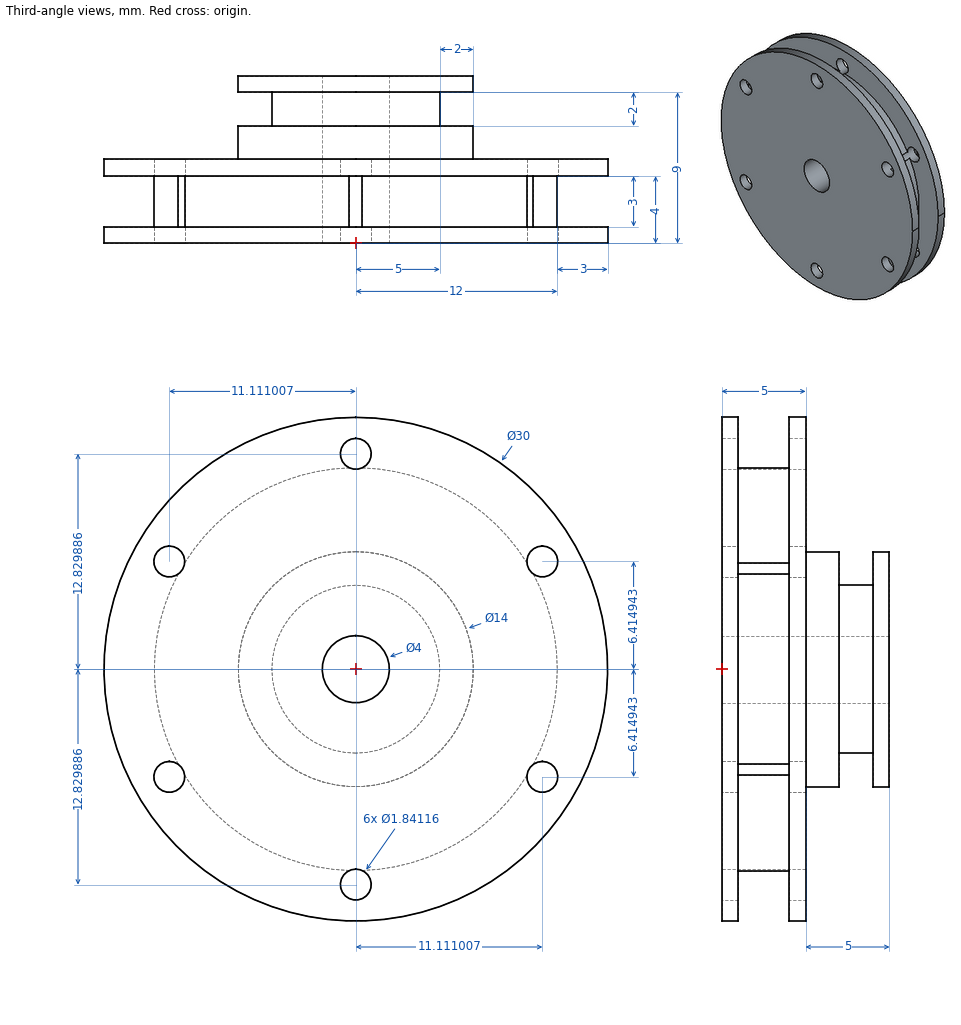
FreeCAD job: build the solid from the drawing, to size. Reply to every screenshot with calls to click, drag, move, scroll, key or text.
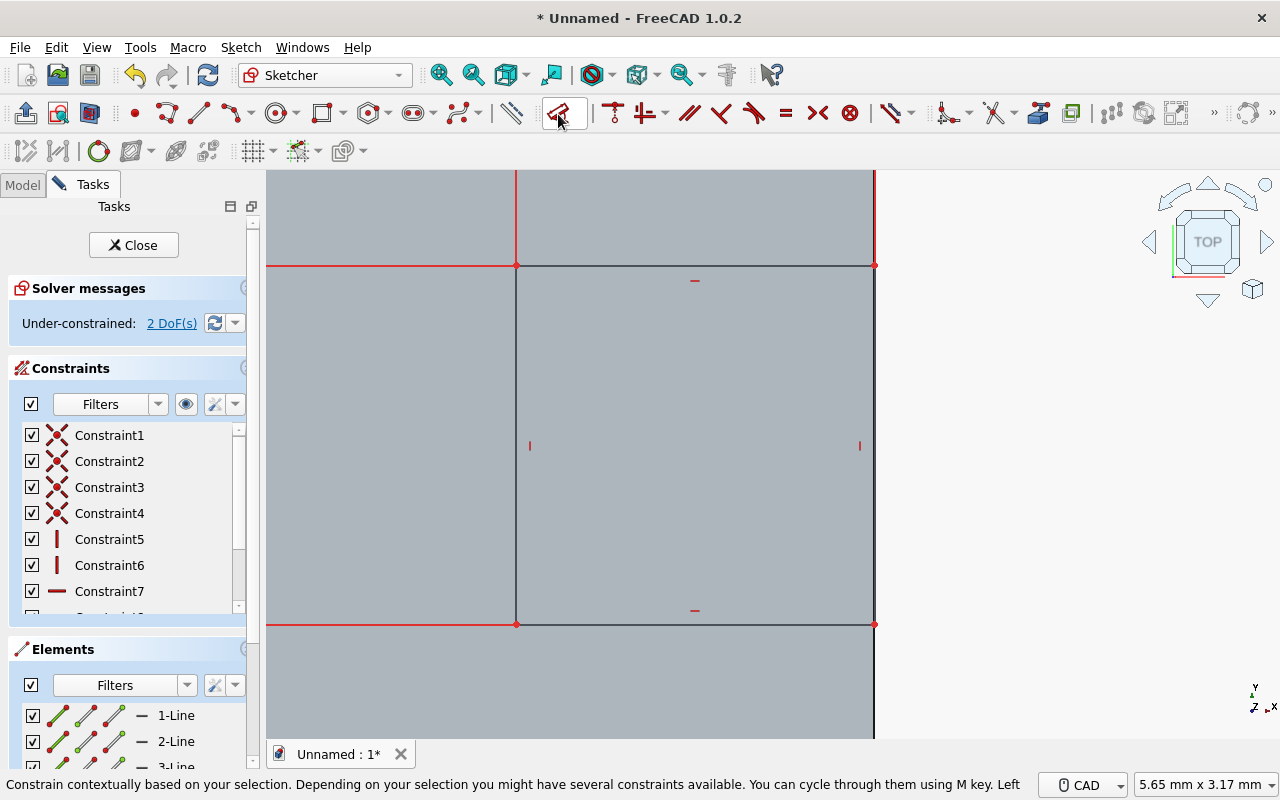
click(516, 266)
click(405, 232)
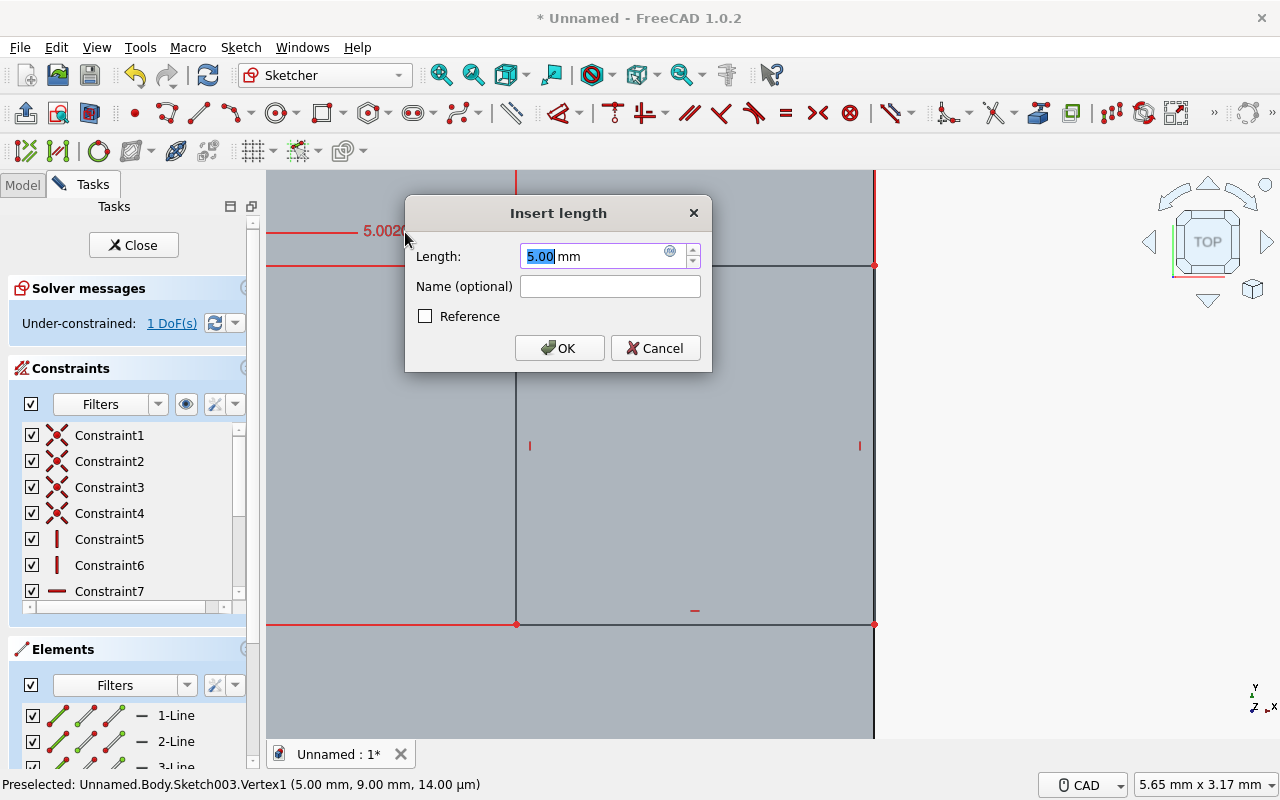
text(5)
key(Return)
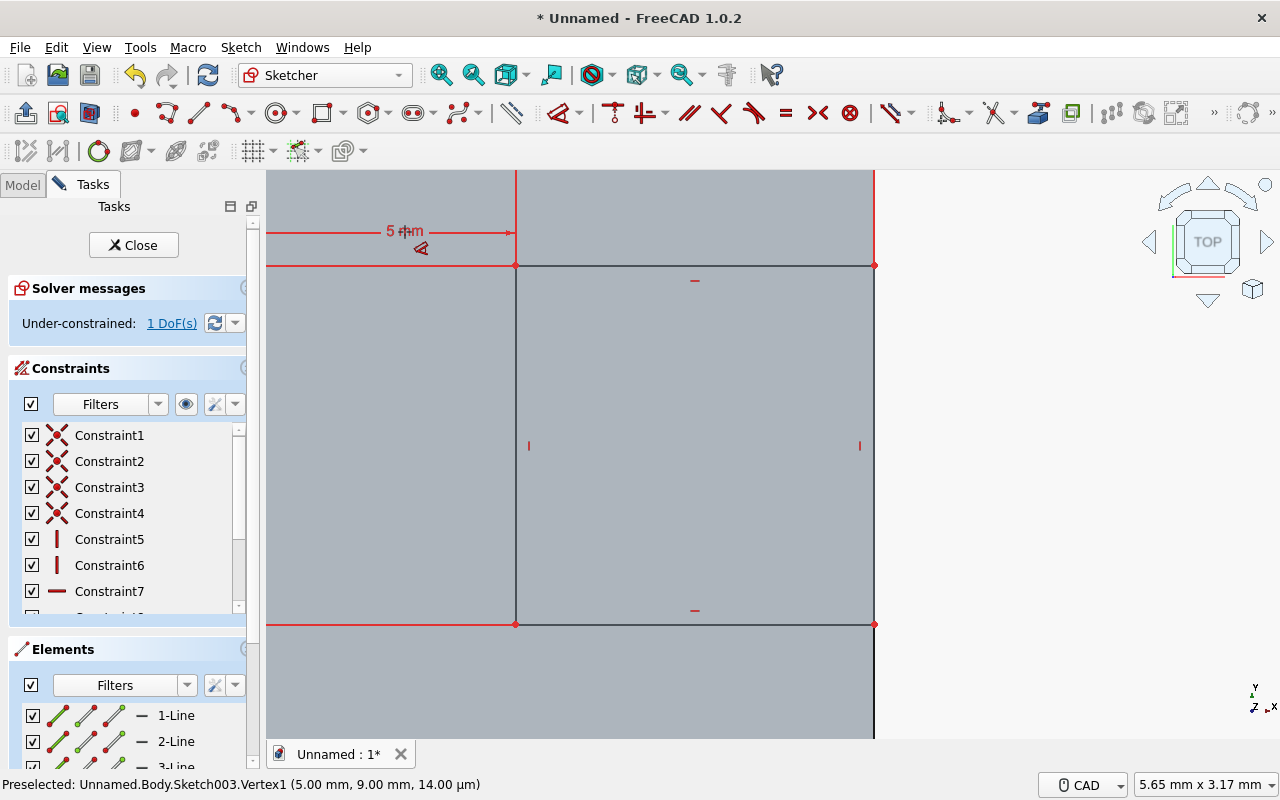
click(516, 266)
click(550, 489)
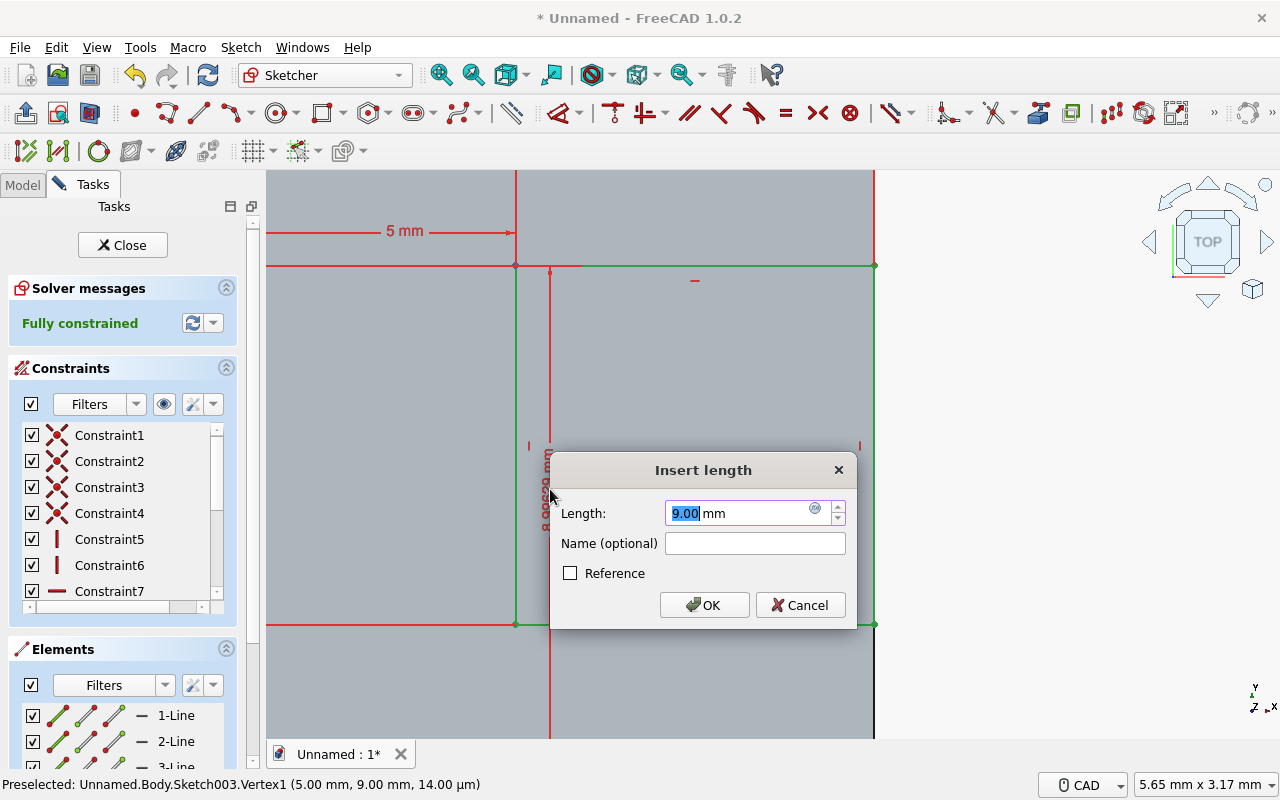
text(9)
key(Return)
key(Escape)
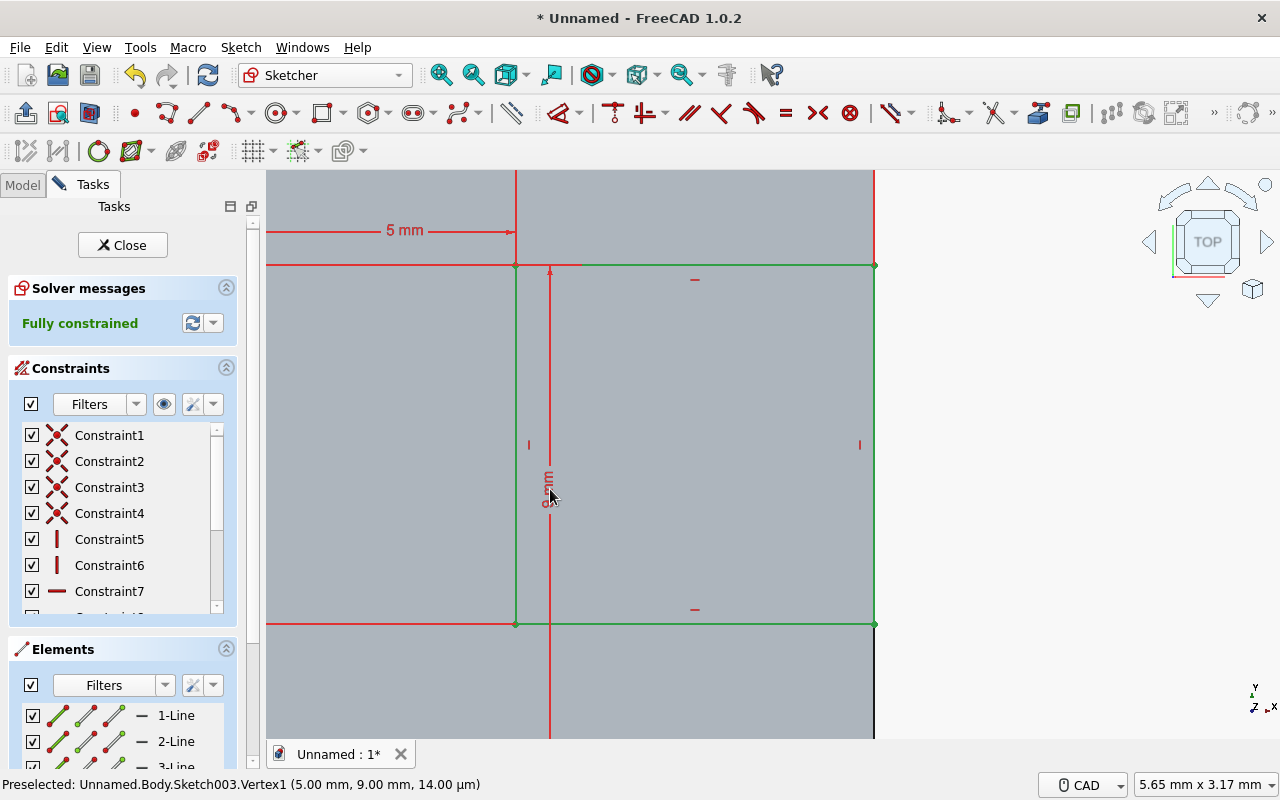
click(123, 245)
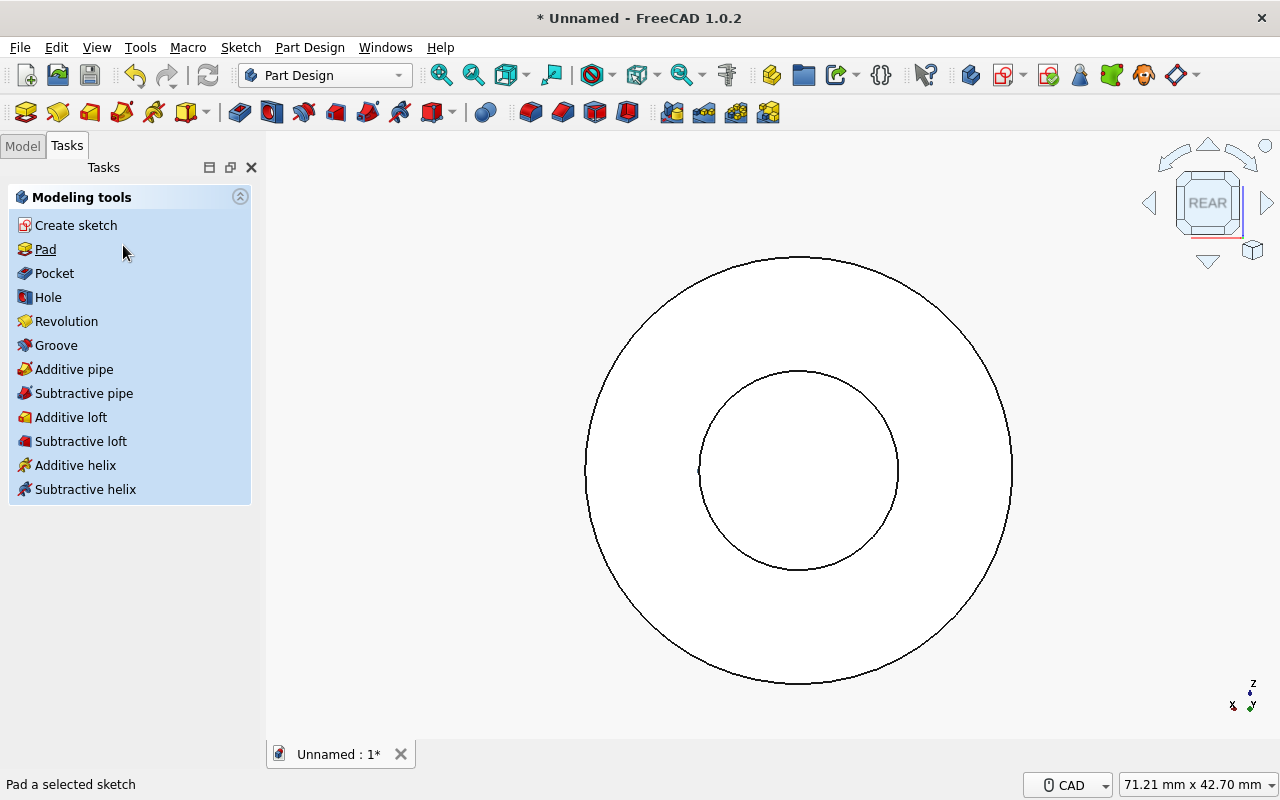
click(304, 112)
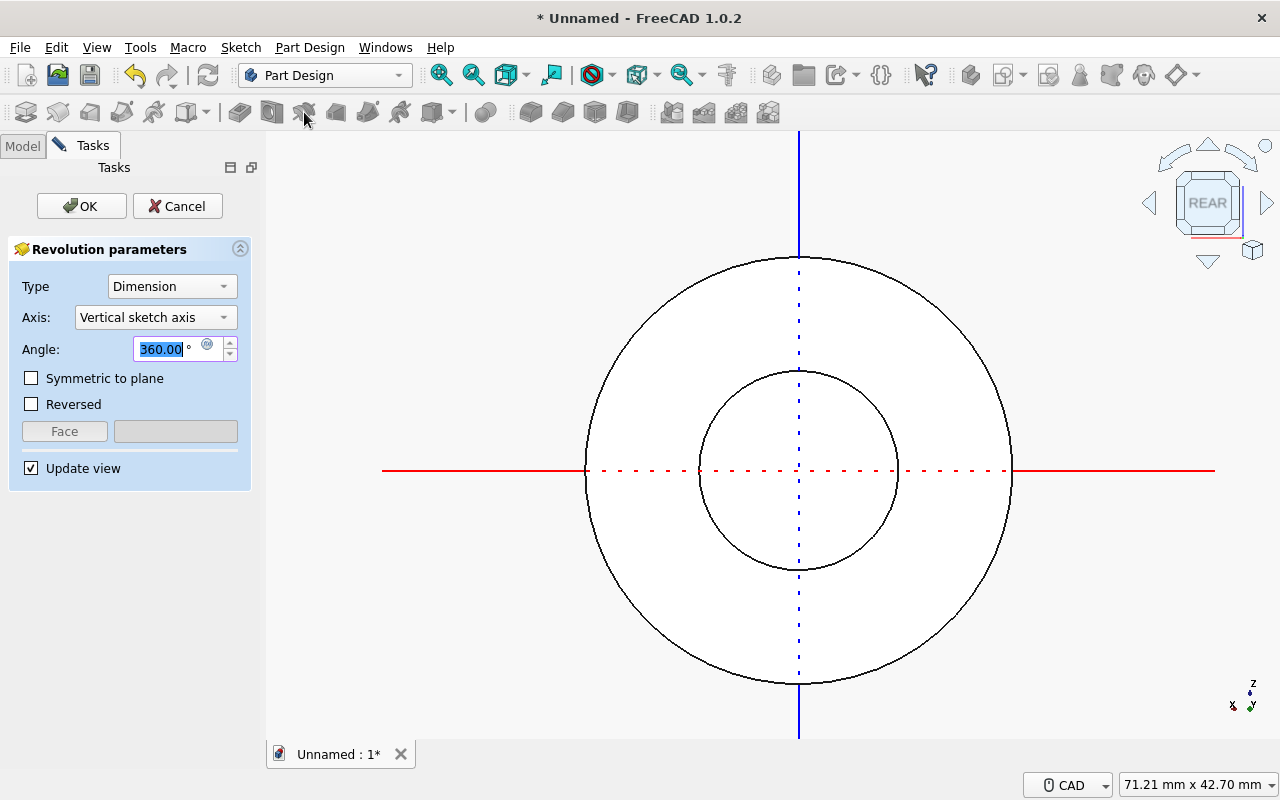
click(82, 206)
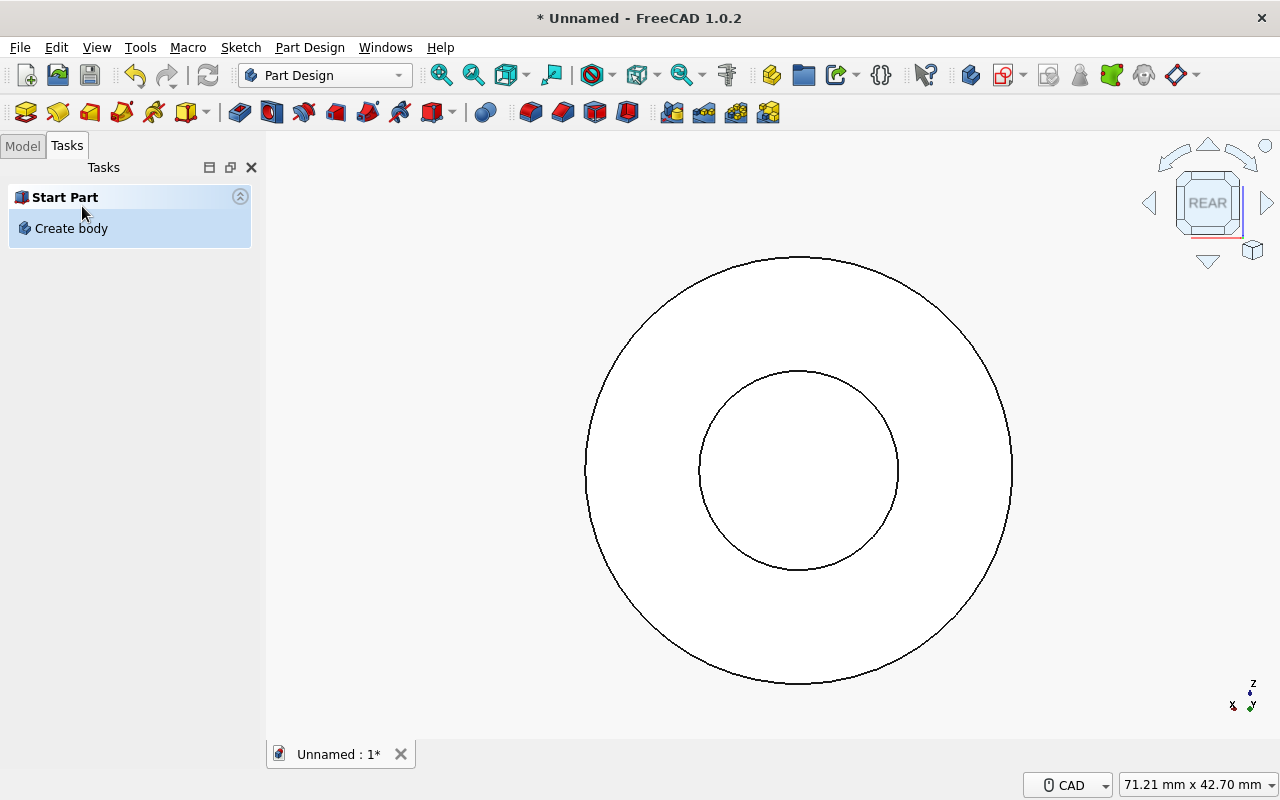
click(799, 470)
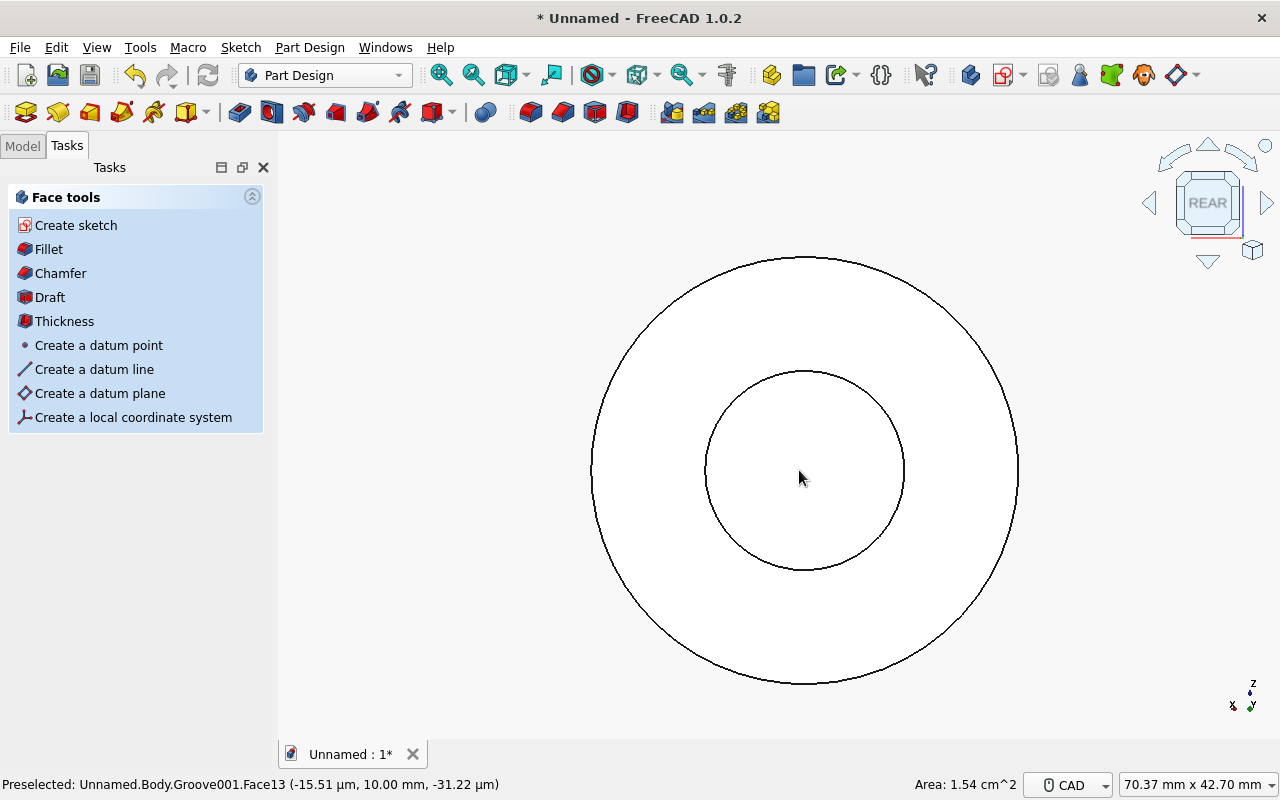
click(1004, 76)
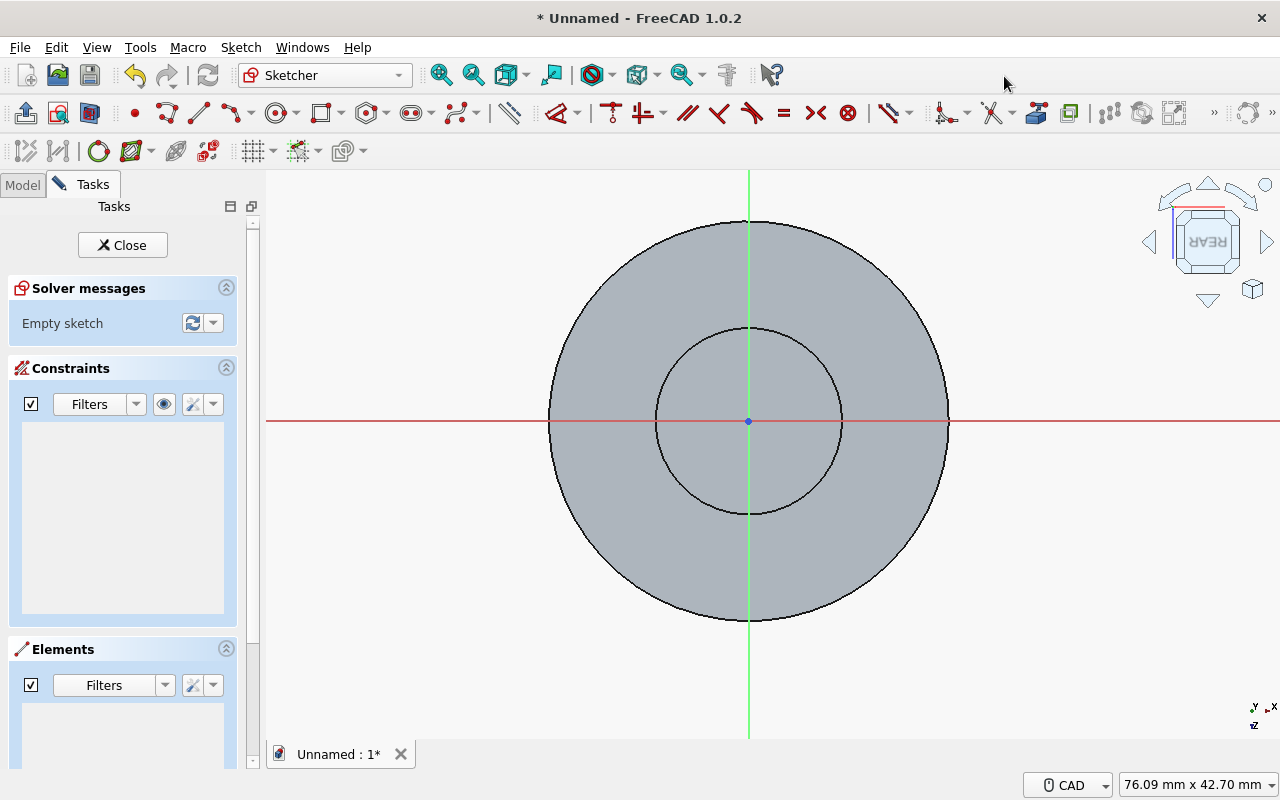
scroll(756, 416, up, 10)